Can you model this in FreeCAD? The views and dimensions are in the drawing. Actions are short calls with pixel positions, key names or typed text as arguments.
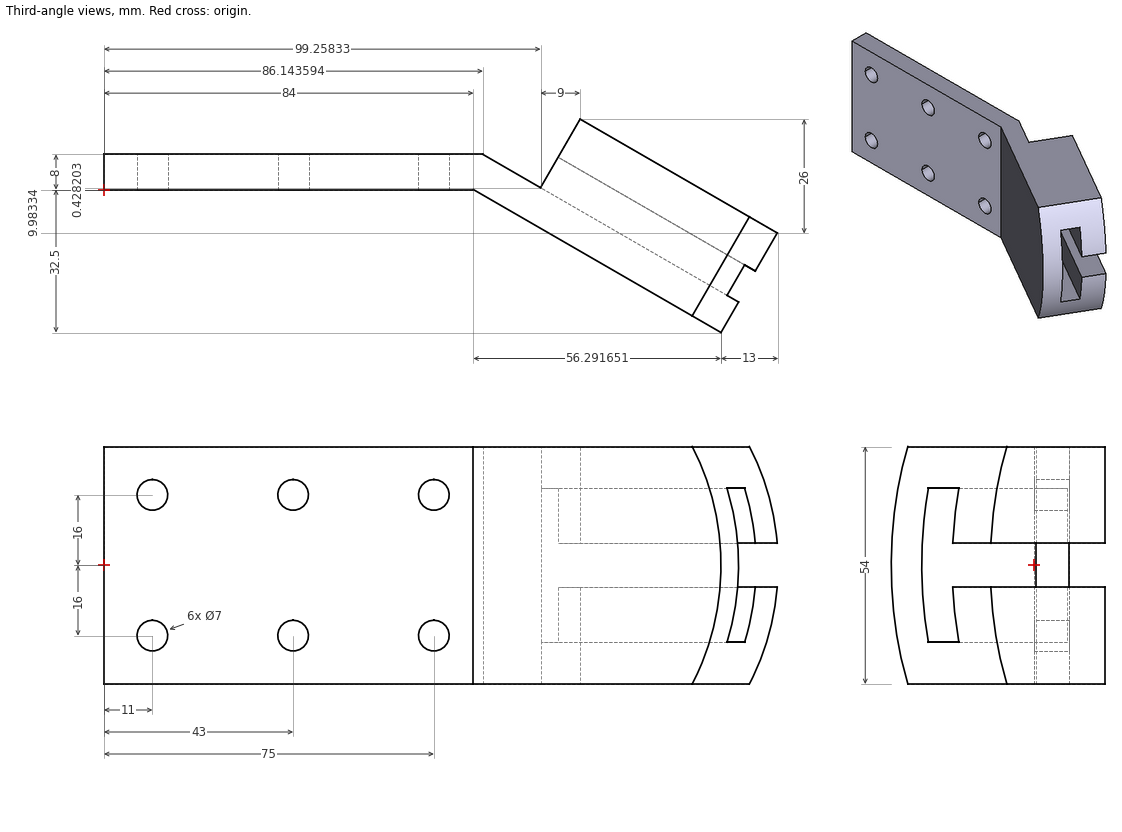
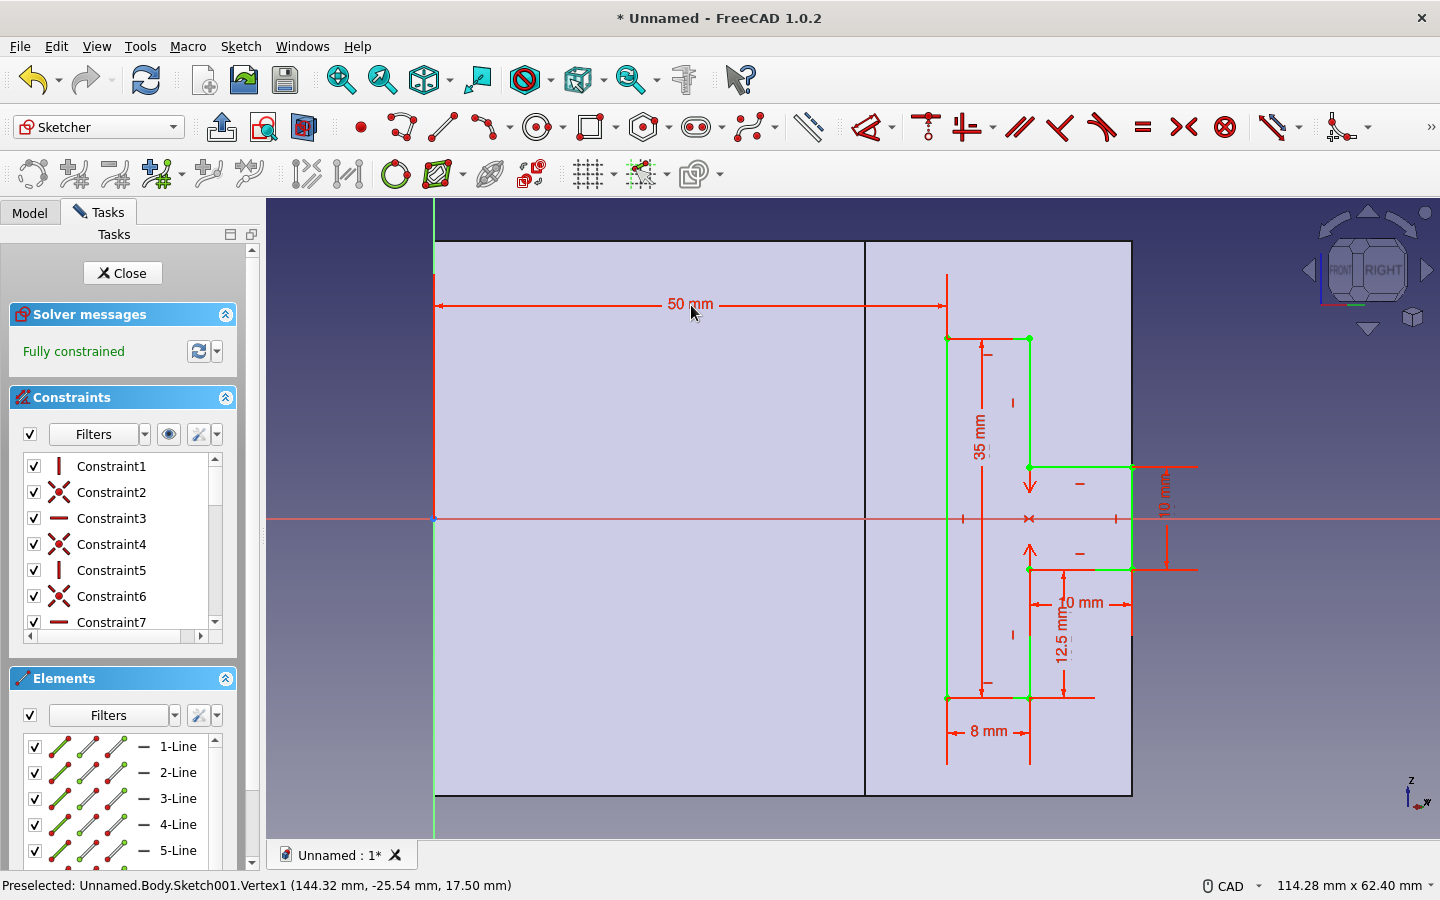
click(123, 273)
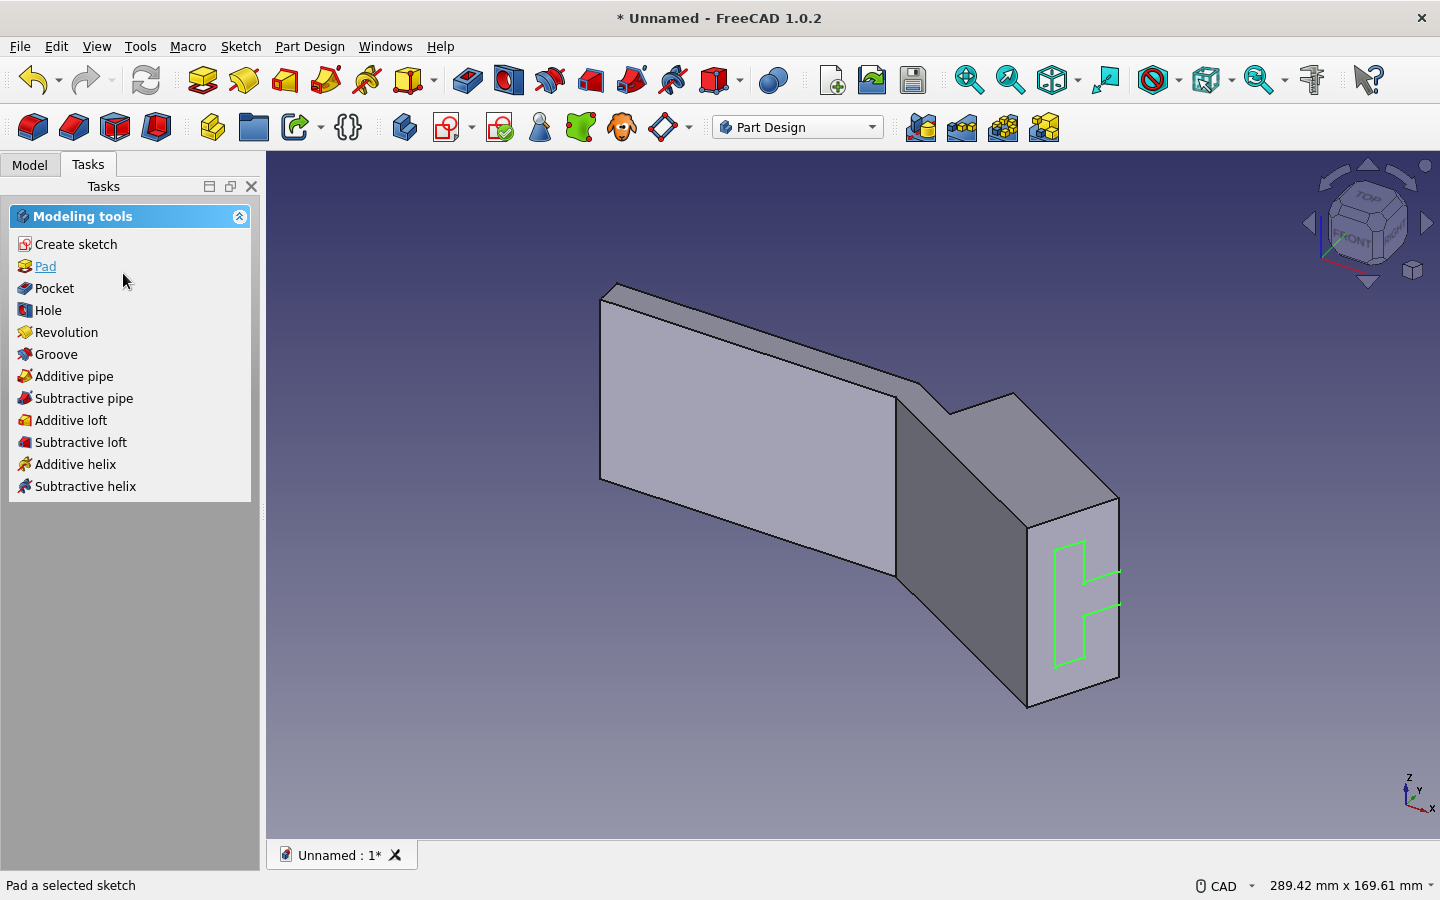
click(468, 80)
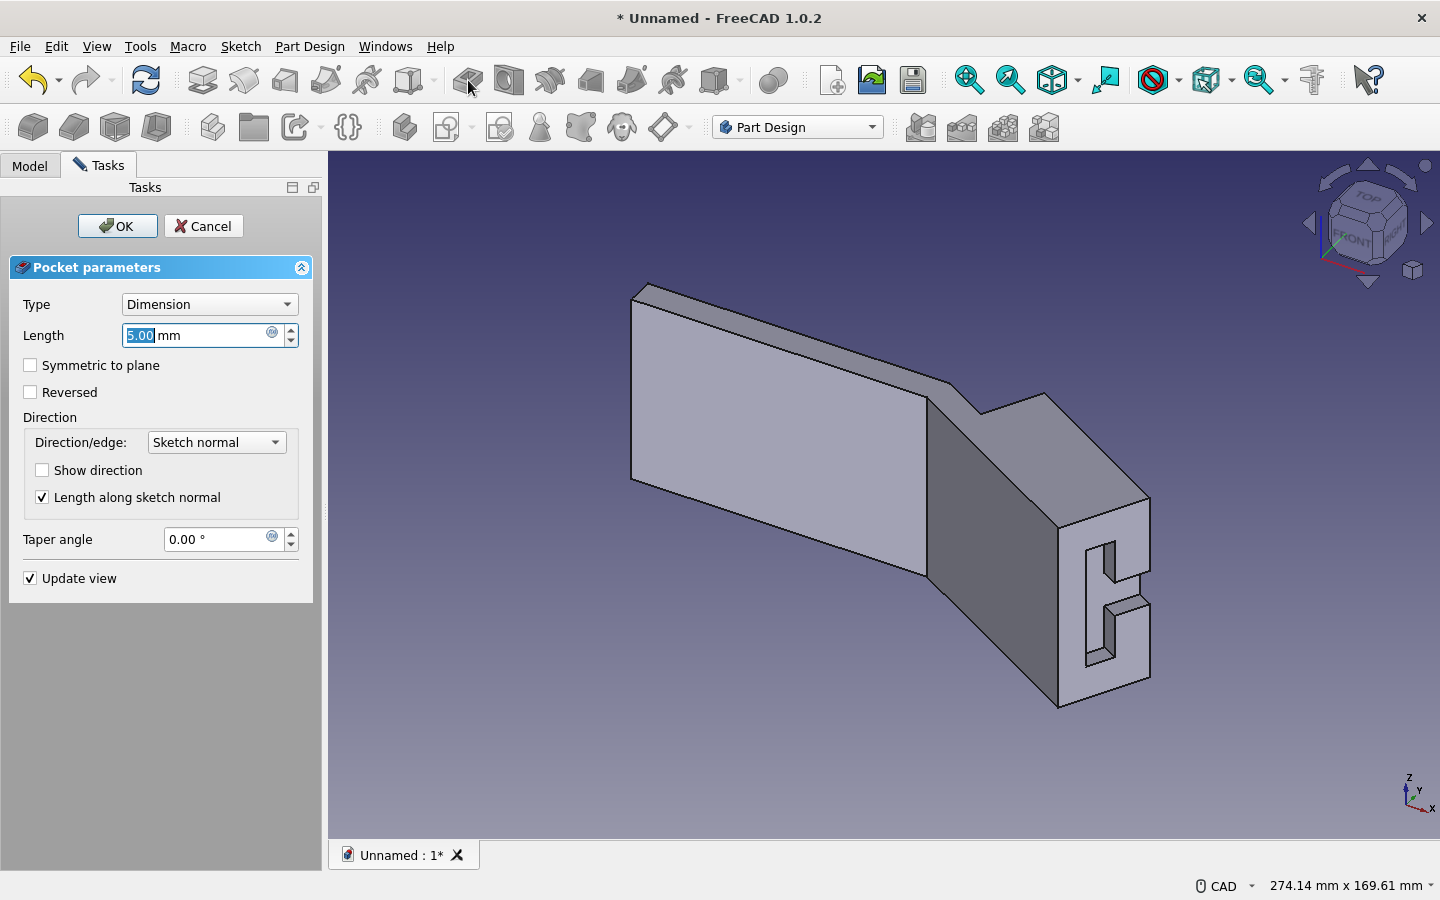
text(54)
key(Tab)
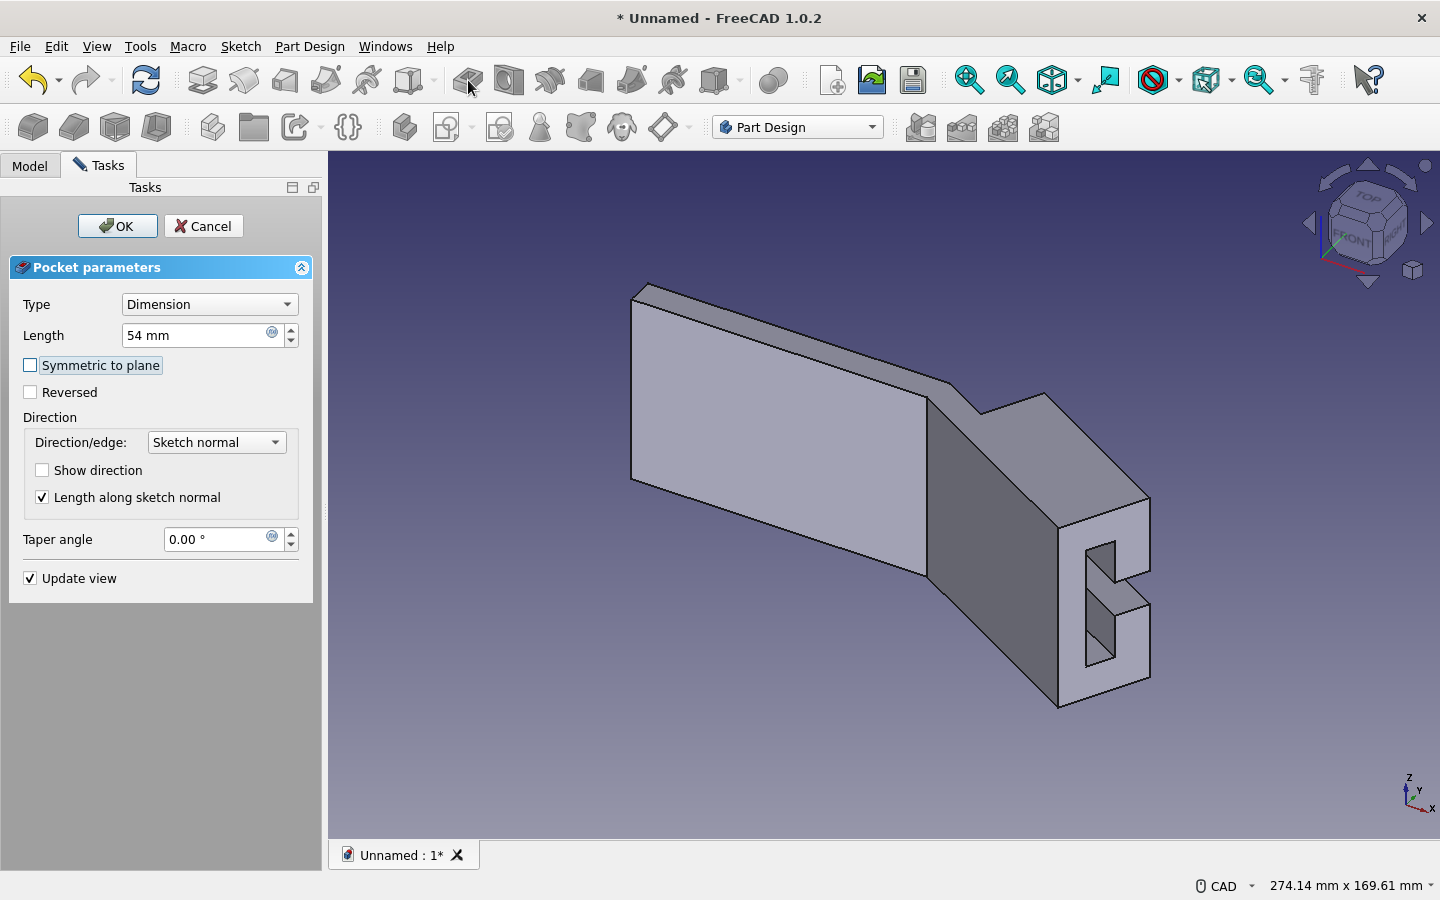
click(118, 226)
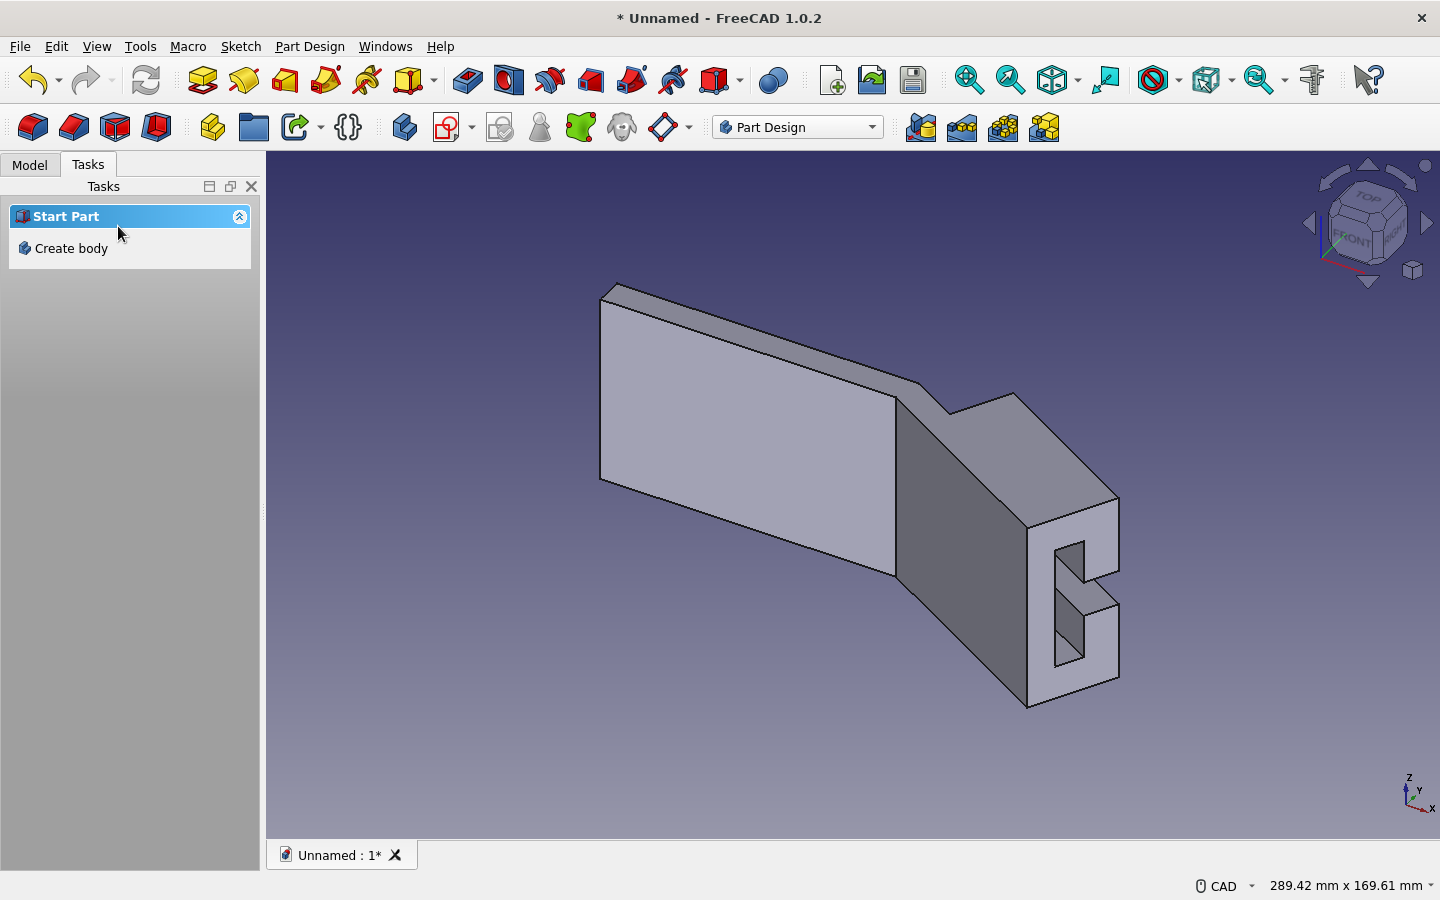
key(4)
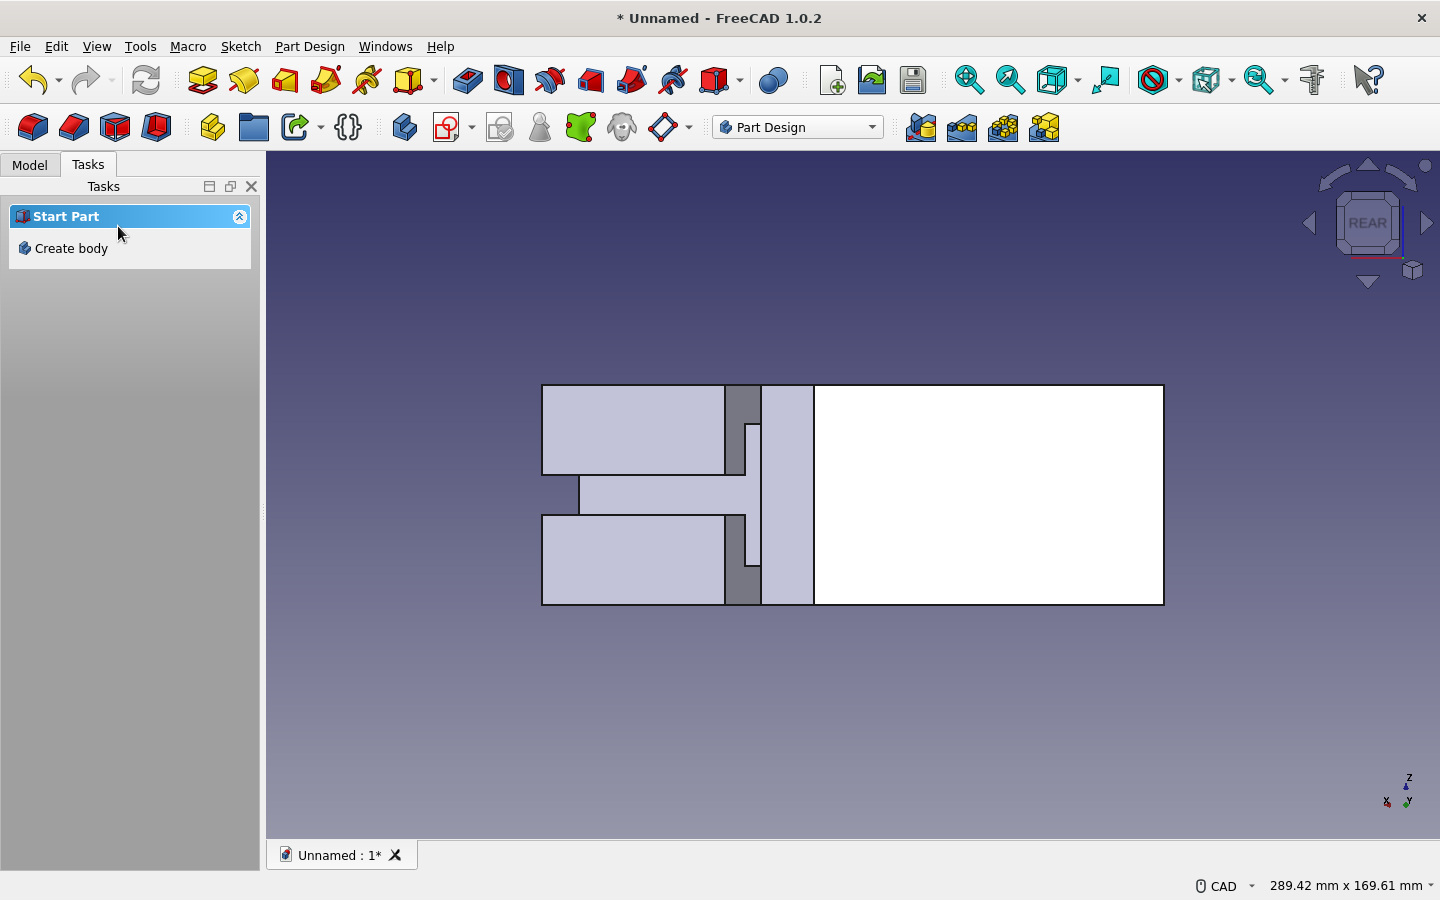
click(581, 559)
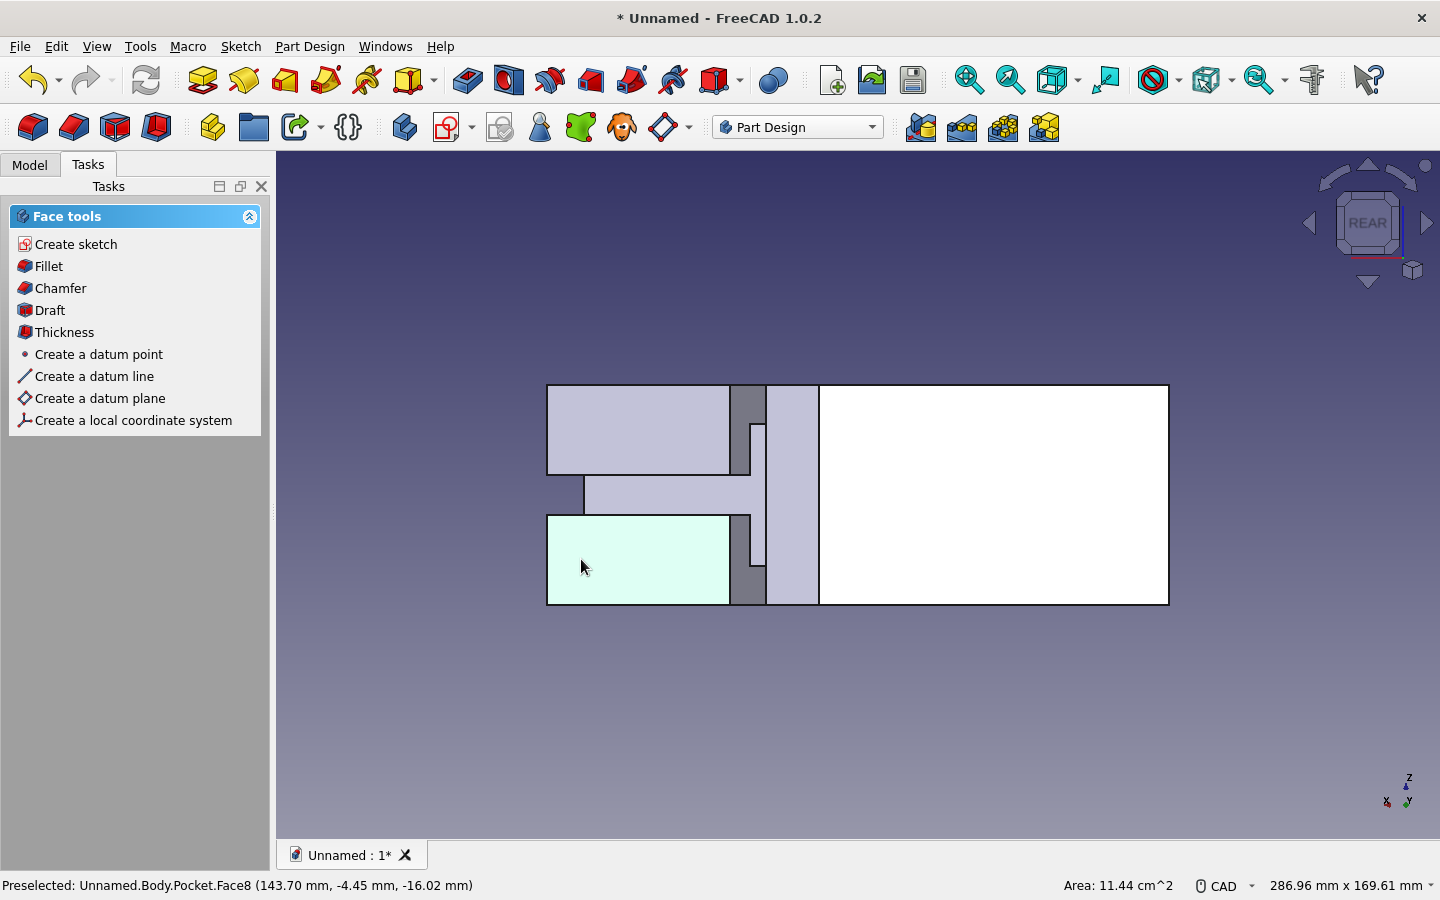
click(446, 128)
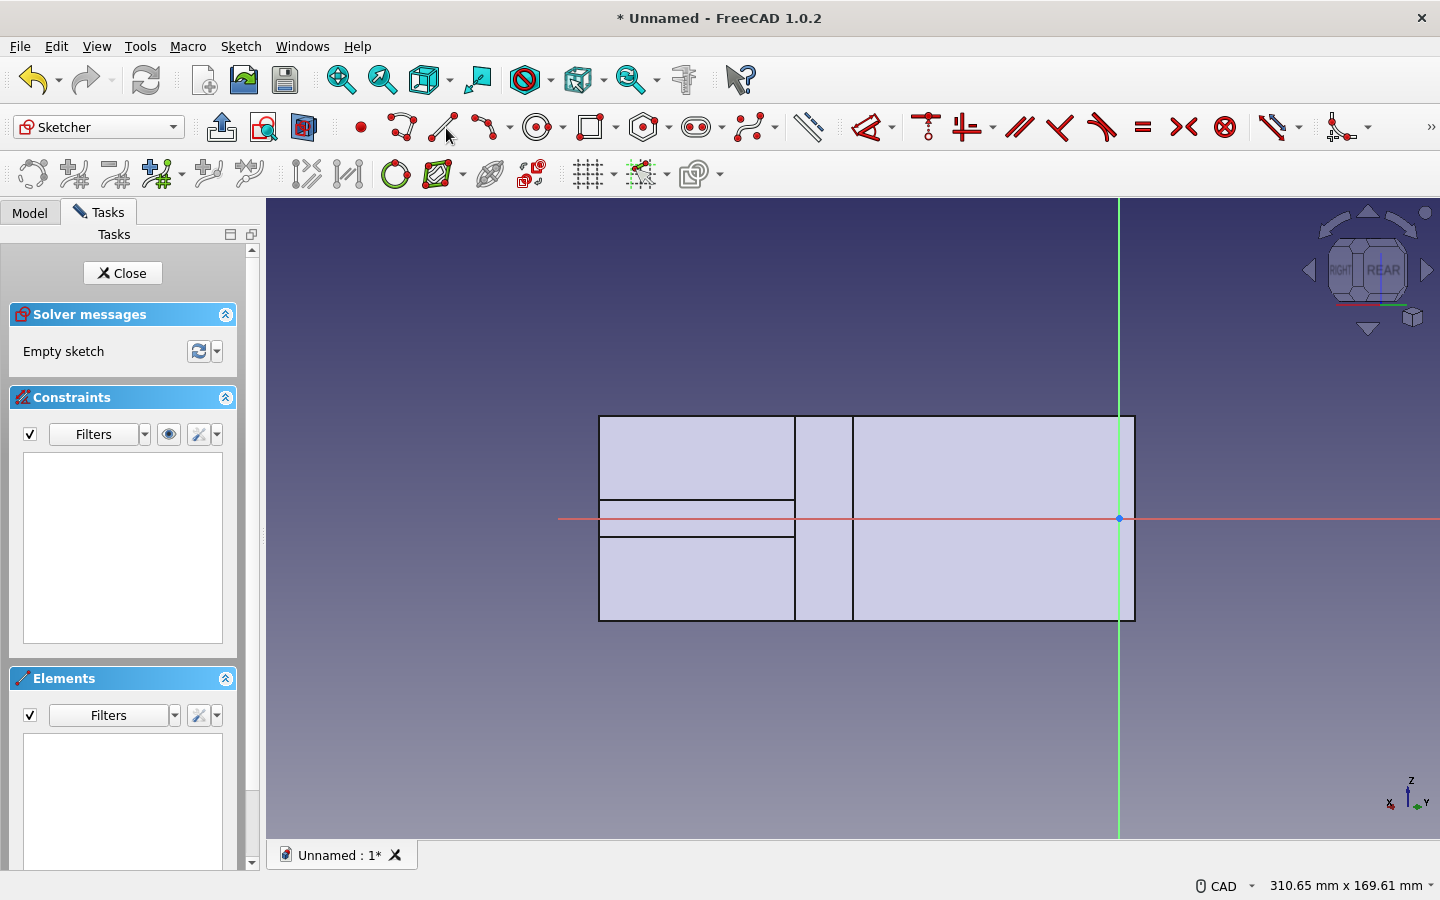
key(q)
key(s)